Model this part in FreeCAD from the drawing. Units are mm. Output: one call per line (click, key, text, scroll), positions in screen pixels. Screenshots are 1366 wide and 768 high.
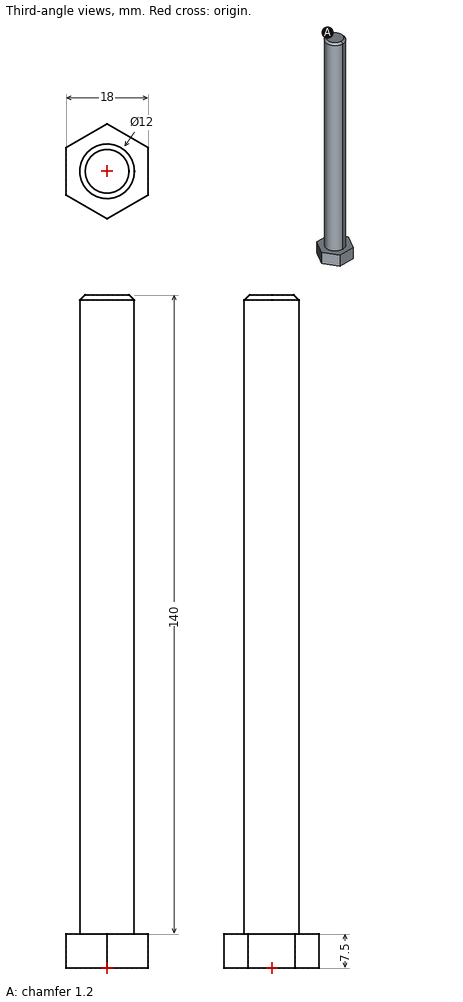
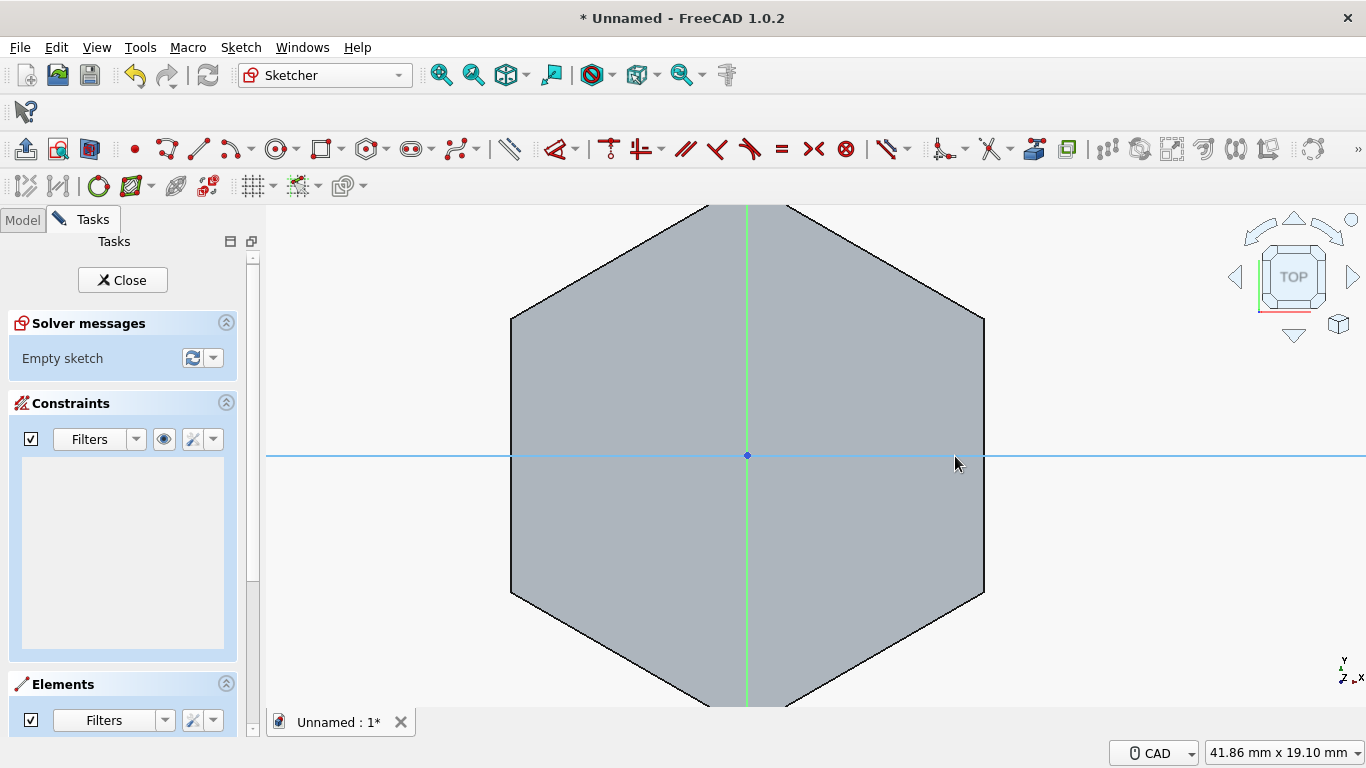
click(276, 150)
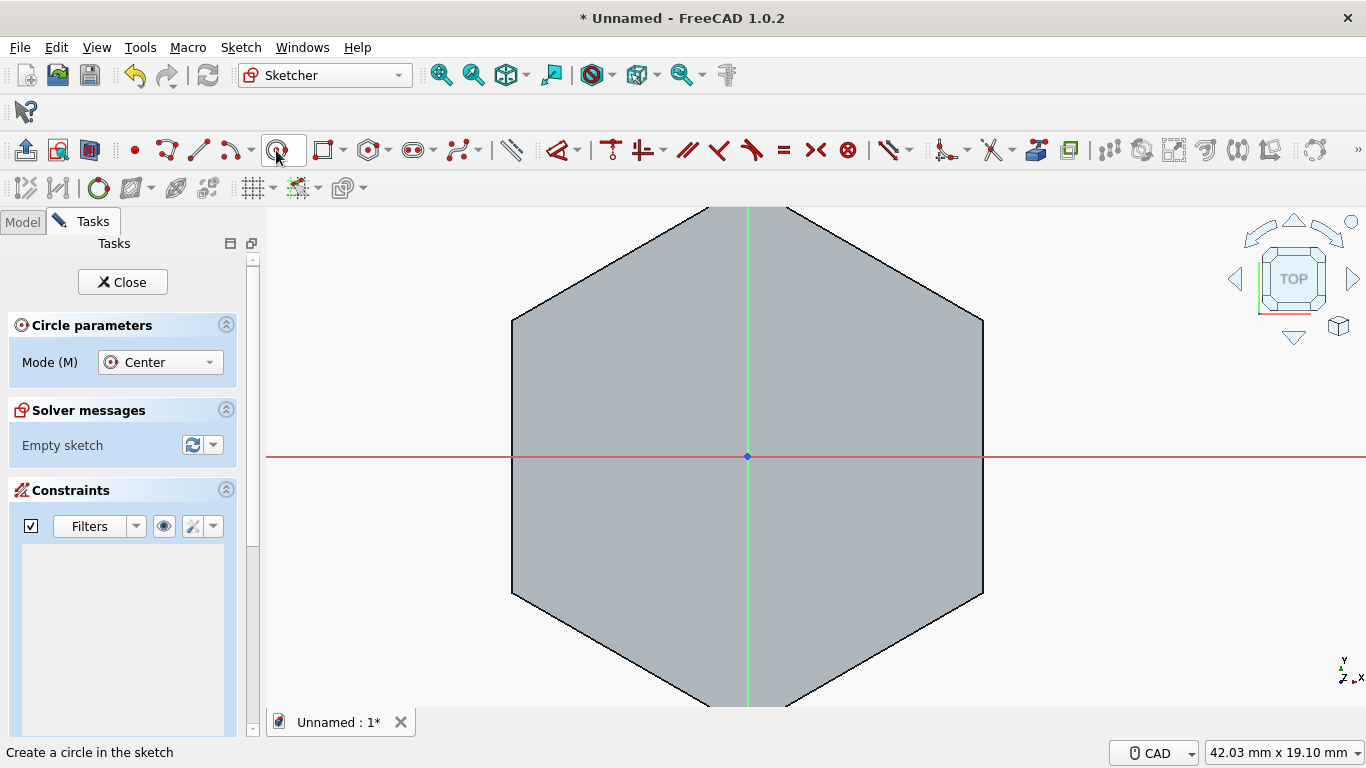
click(748, 457)
move(859, 346)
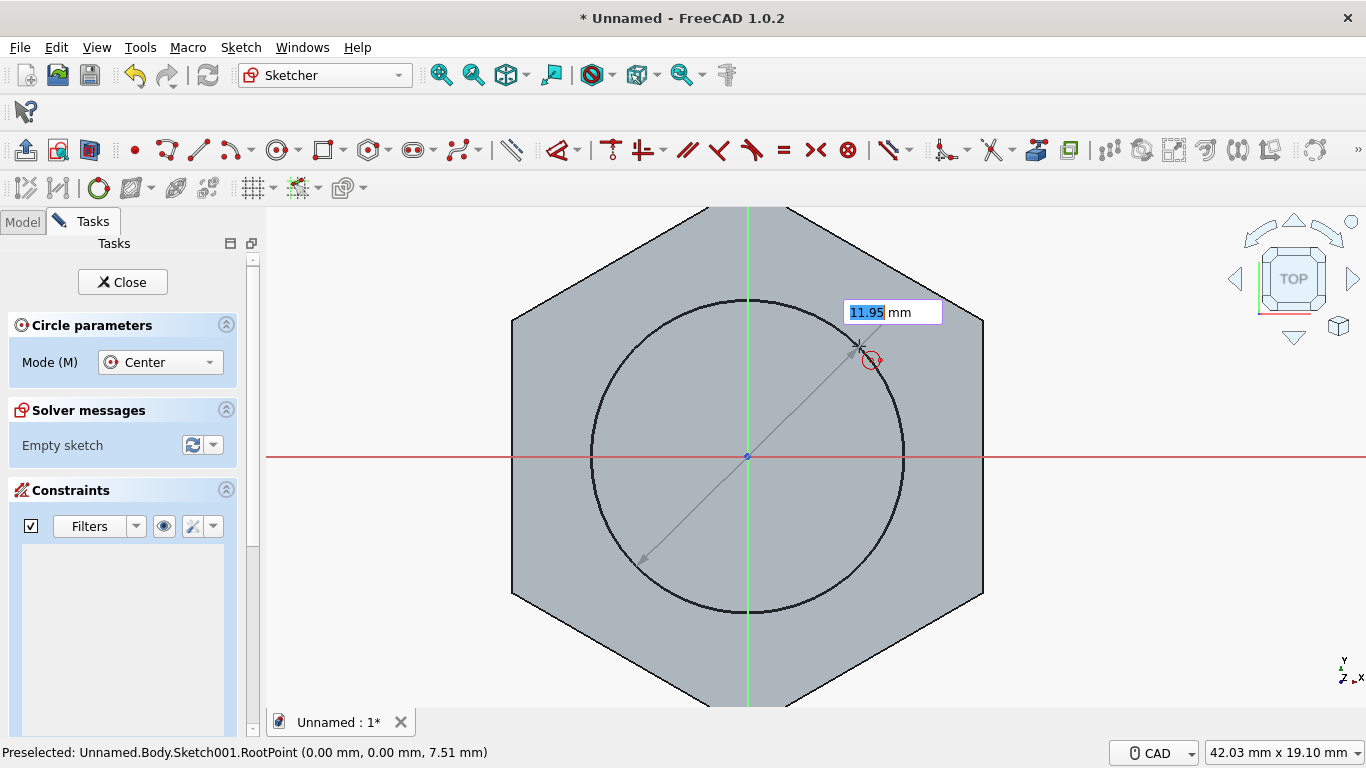
text(12)
key(Return)
key(Escape)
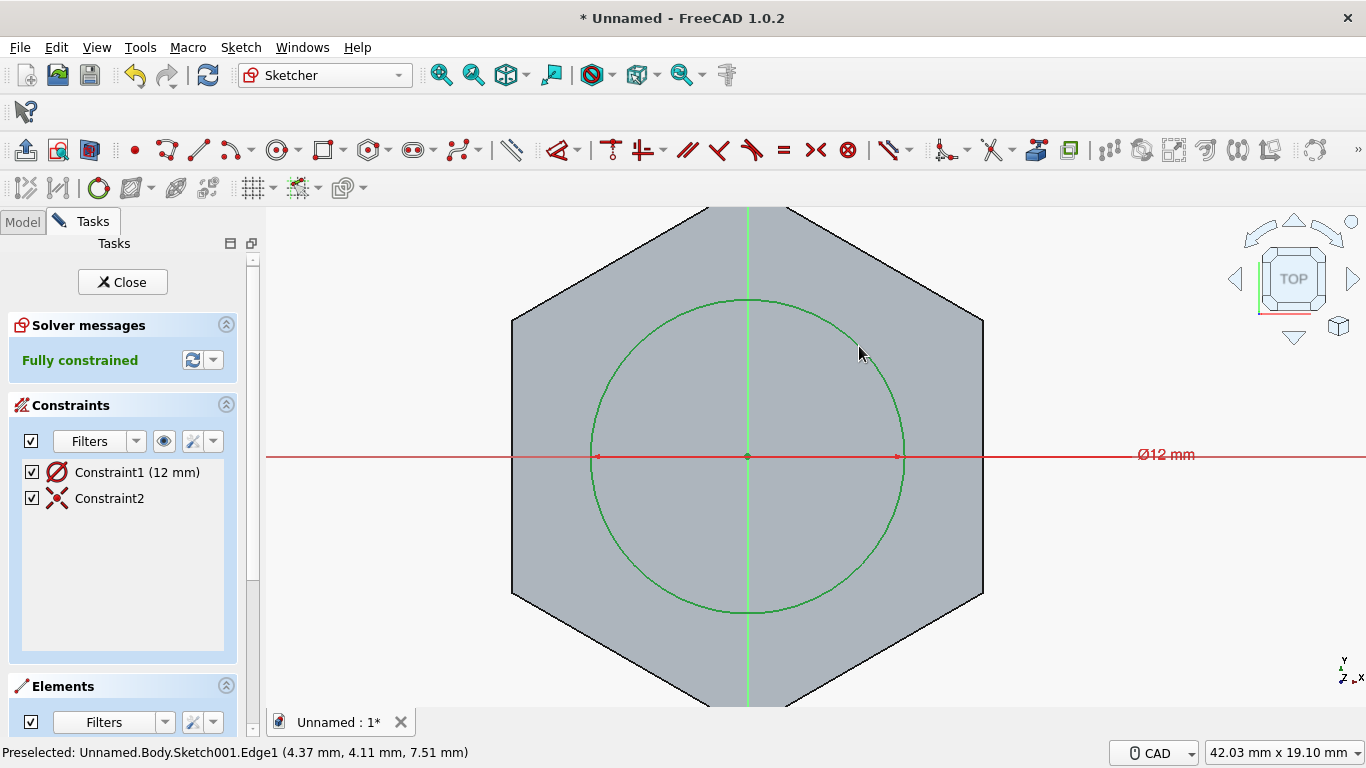
click(123, 282)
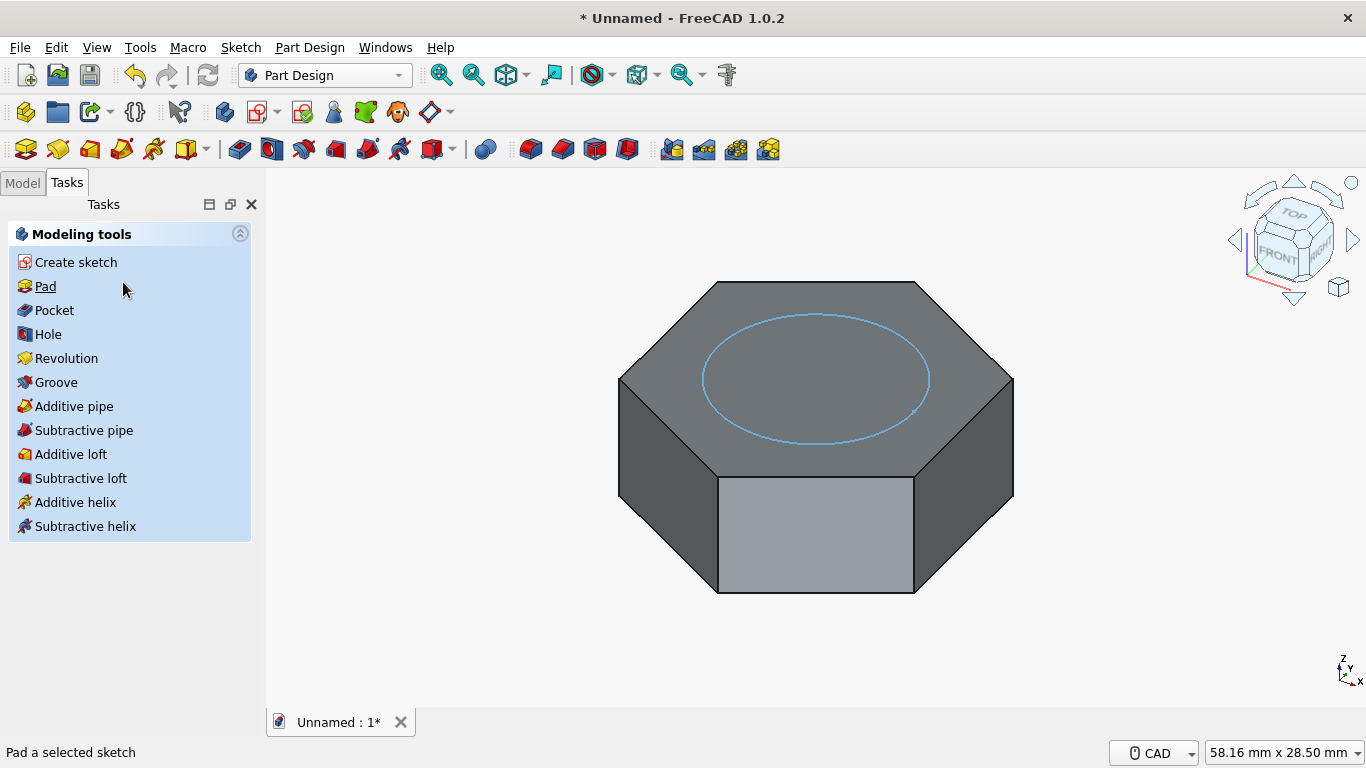
click(26, 150)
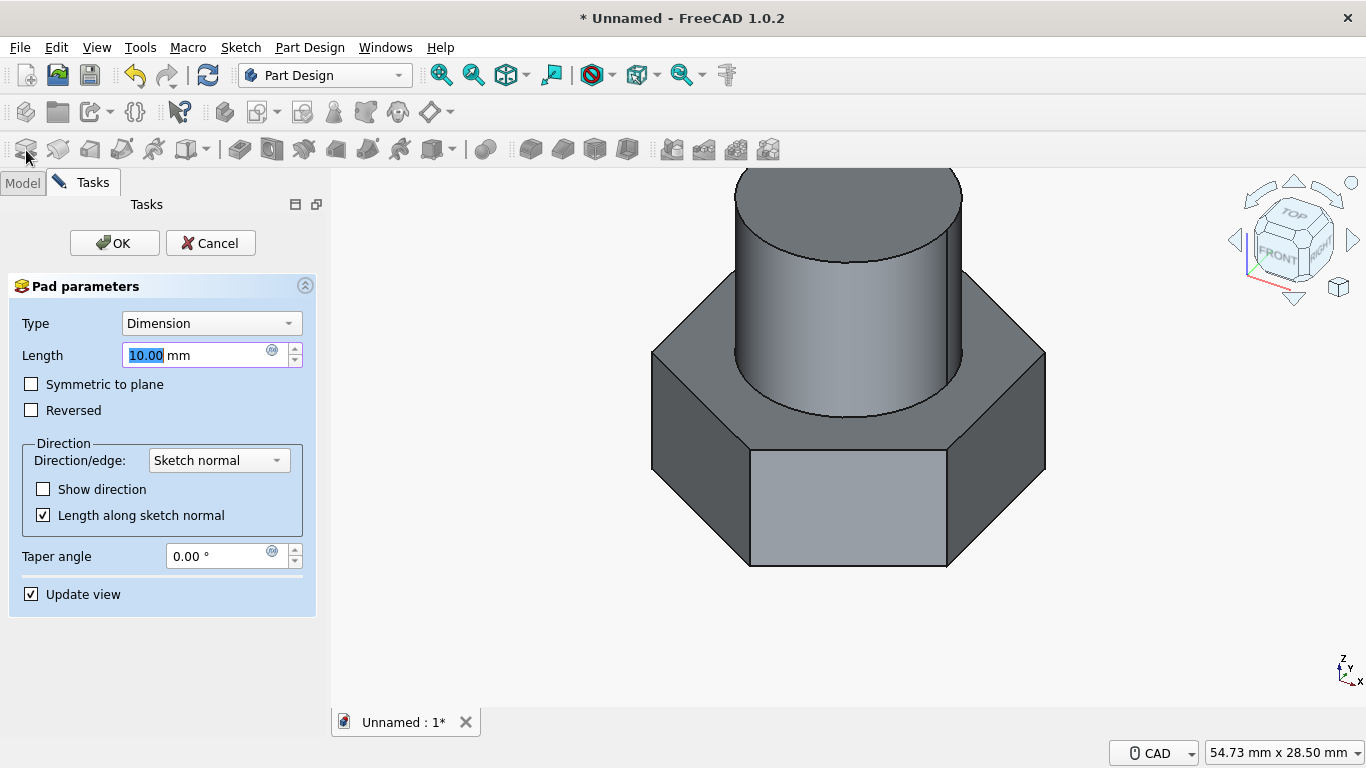
text(140)
key(Tab)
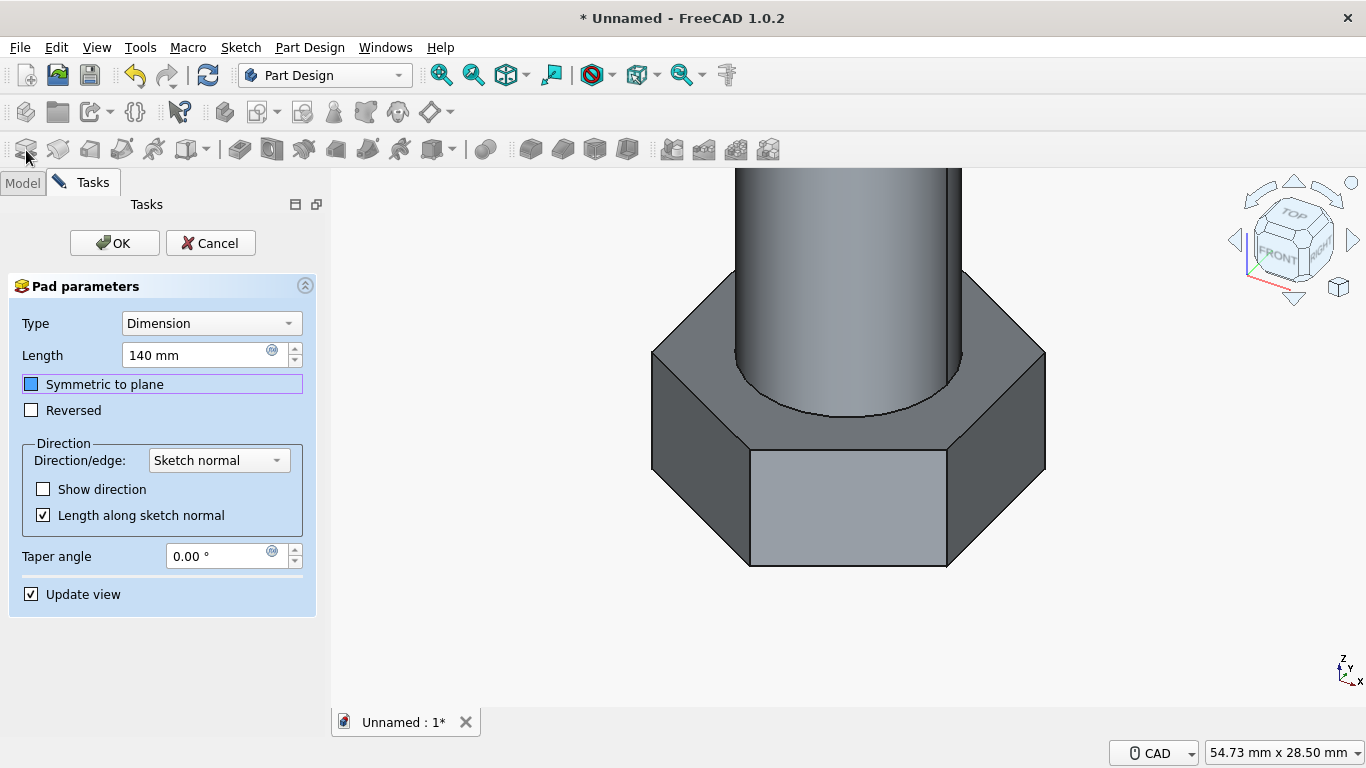
click(115, 243)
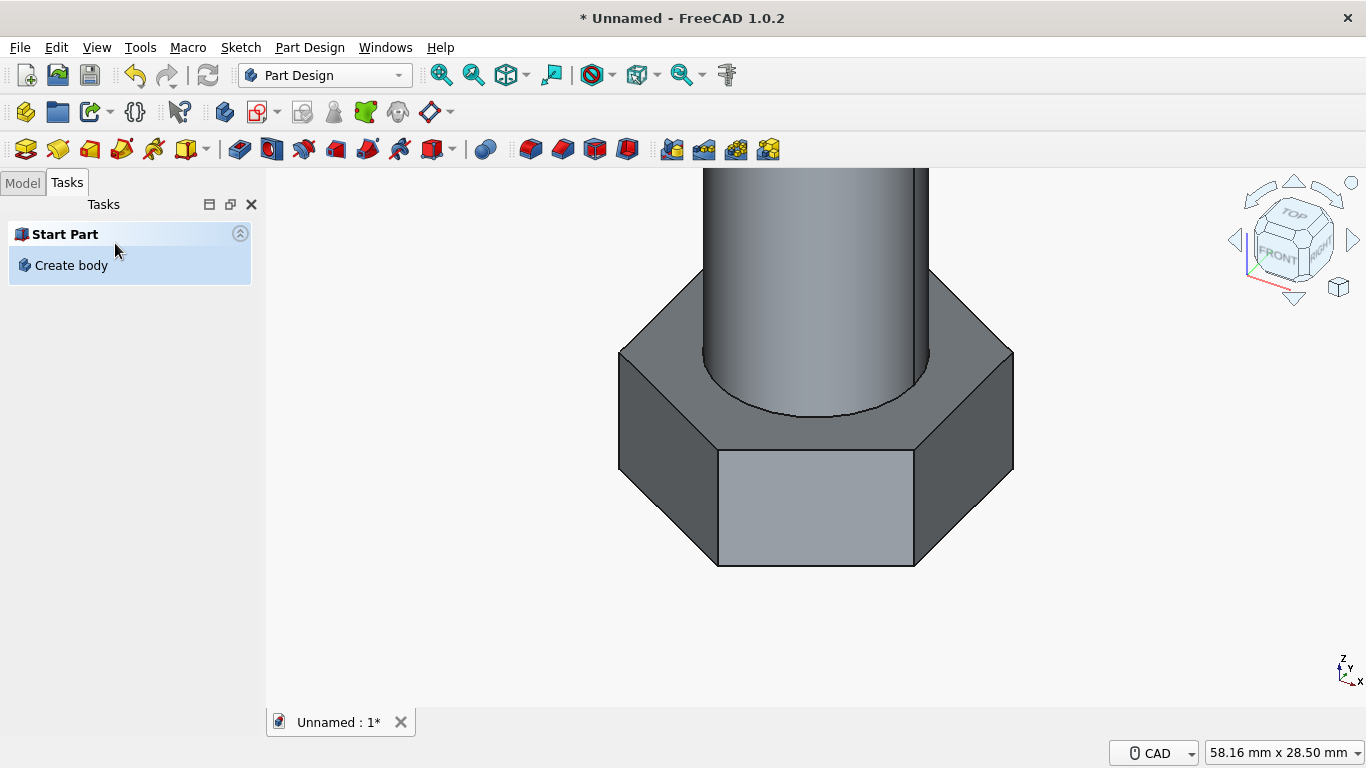
click(442, 76)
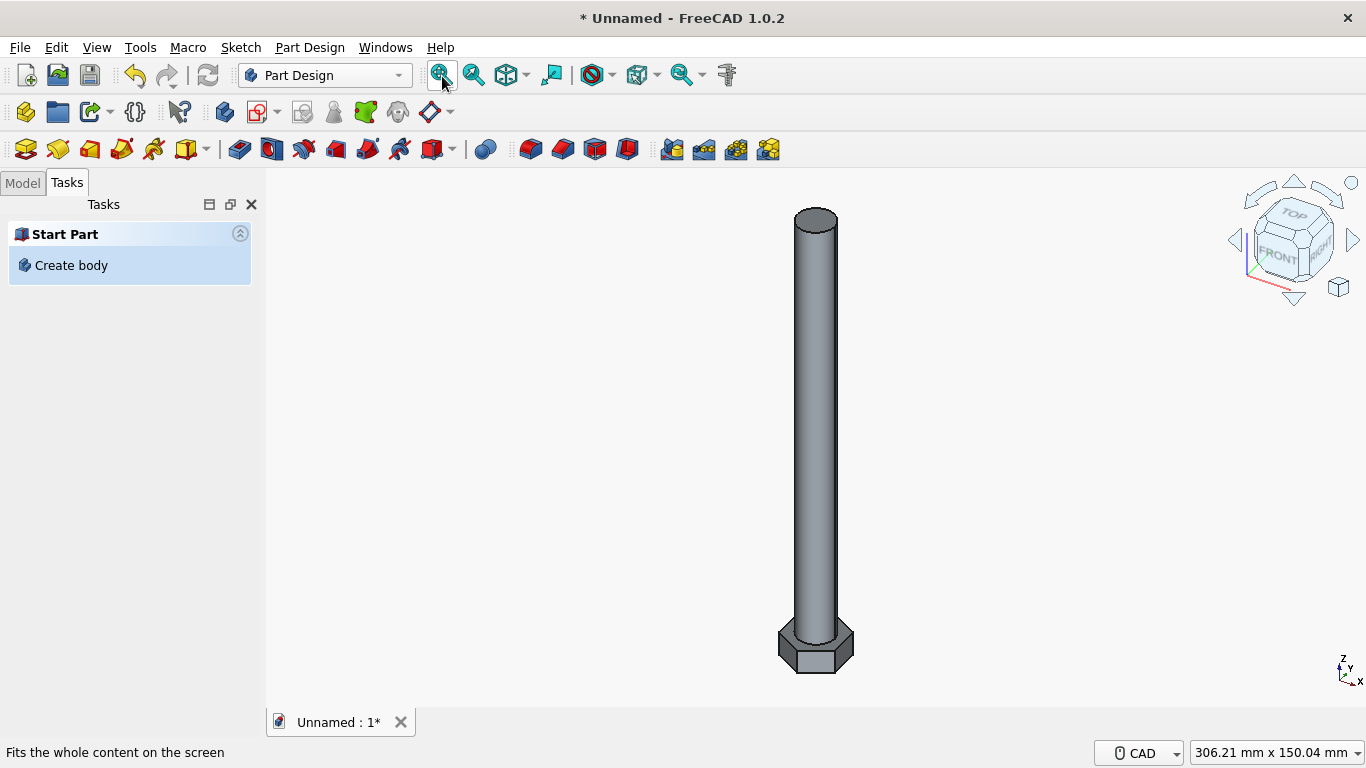
click(807, 208)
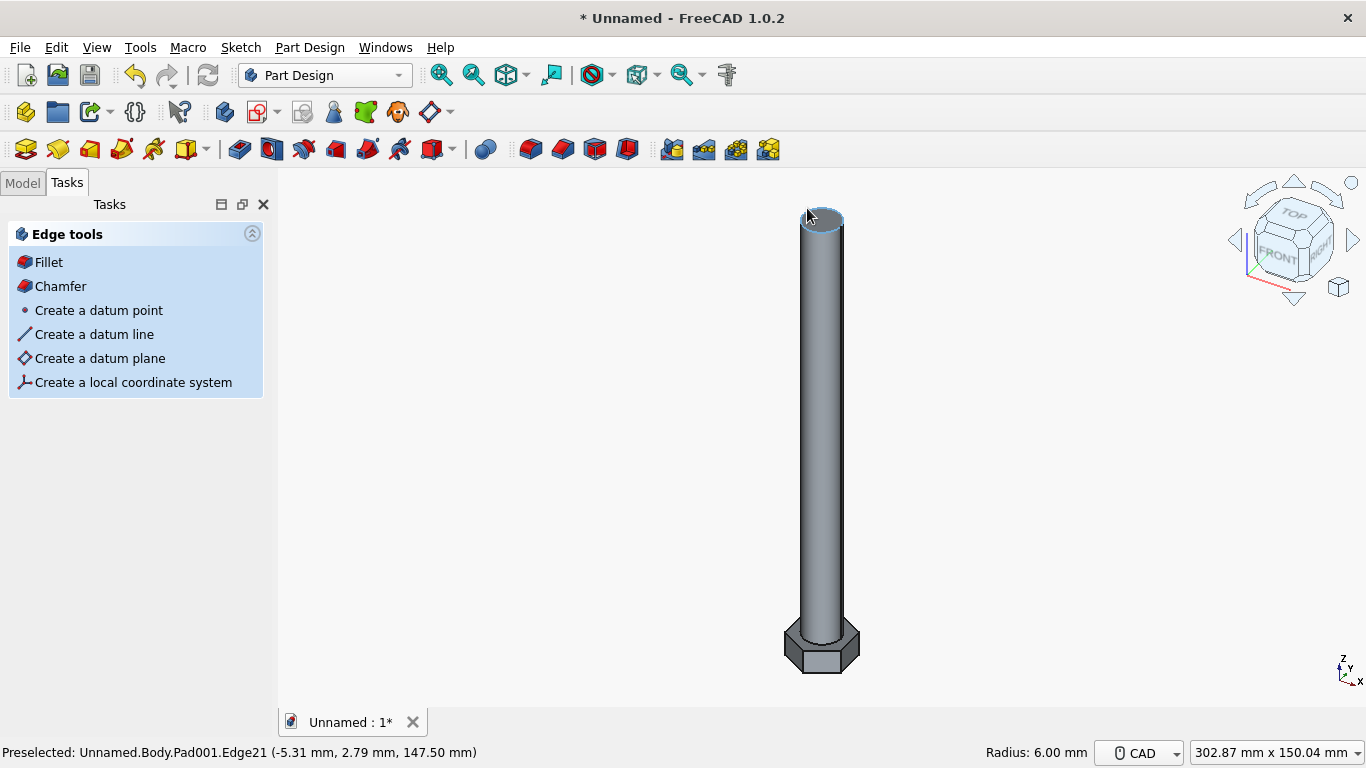
click(564, 150)